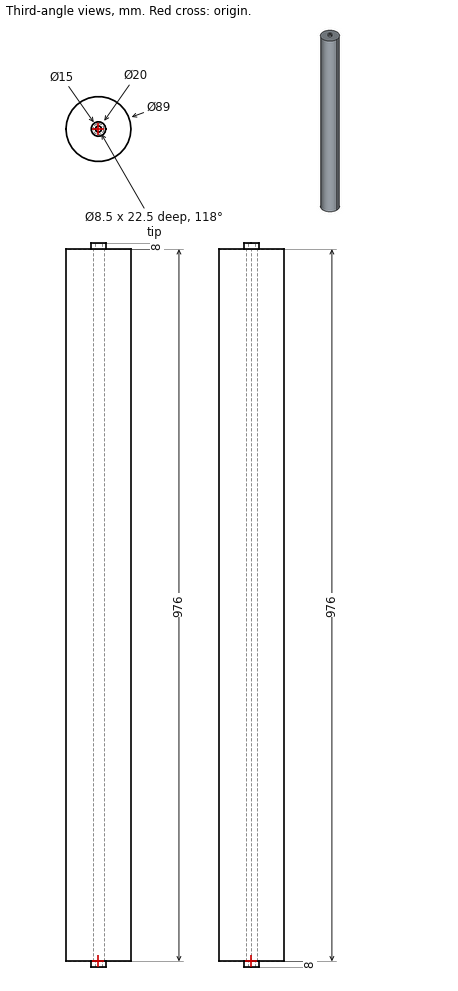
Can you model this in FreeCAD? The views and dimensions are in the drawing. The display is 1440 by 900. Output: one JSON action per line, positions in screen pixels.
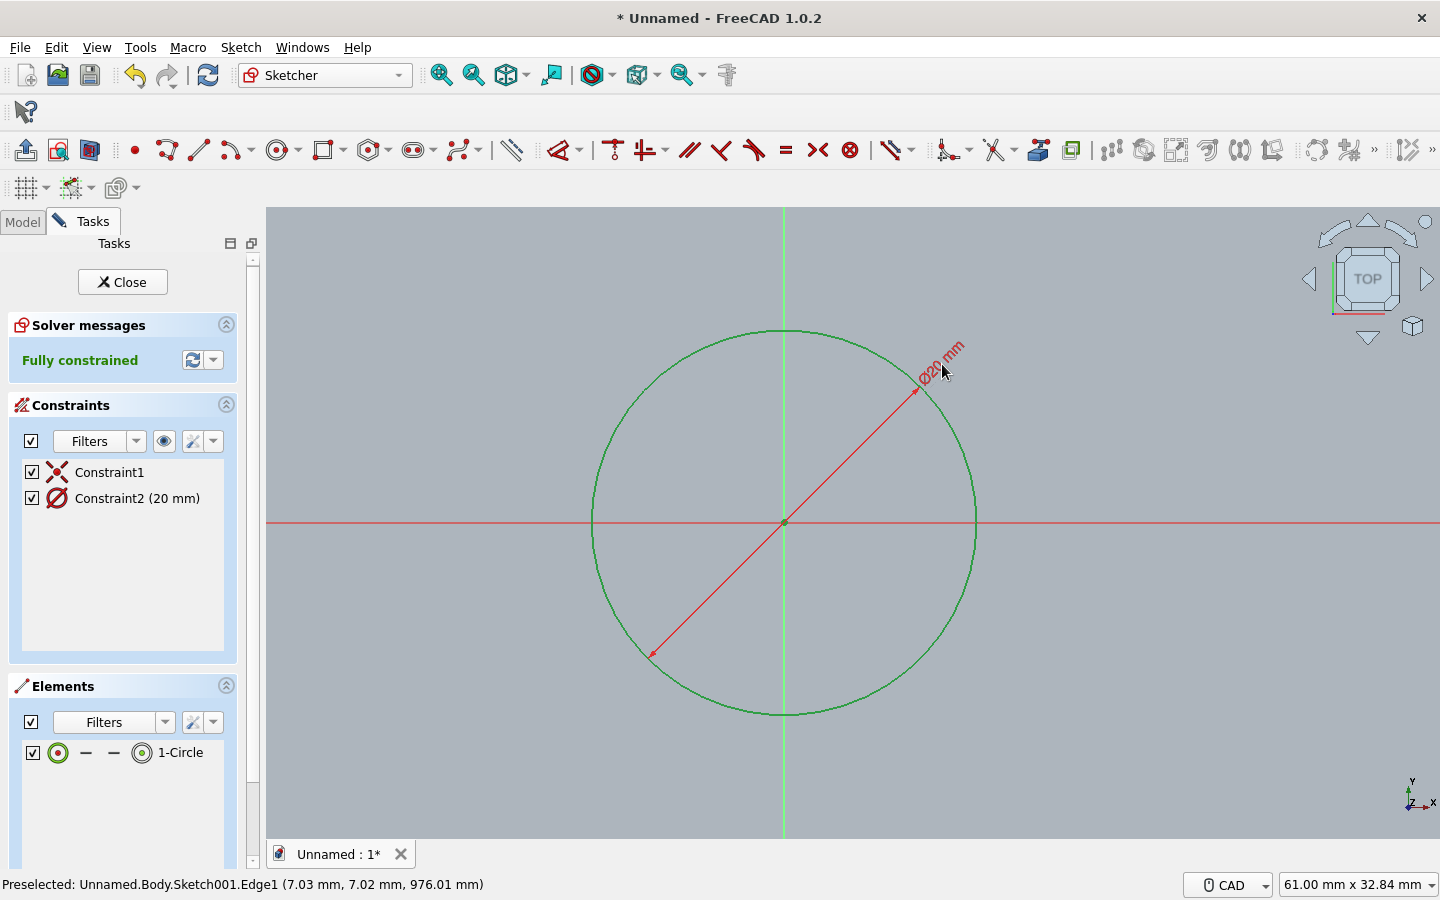
{"action": "left_click", "coordinate": [123, 282]}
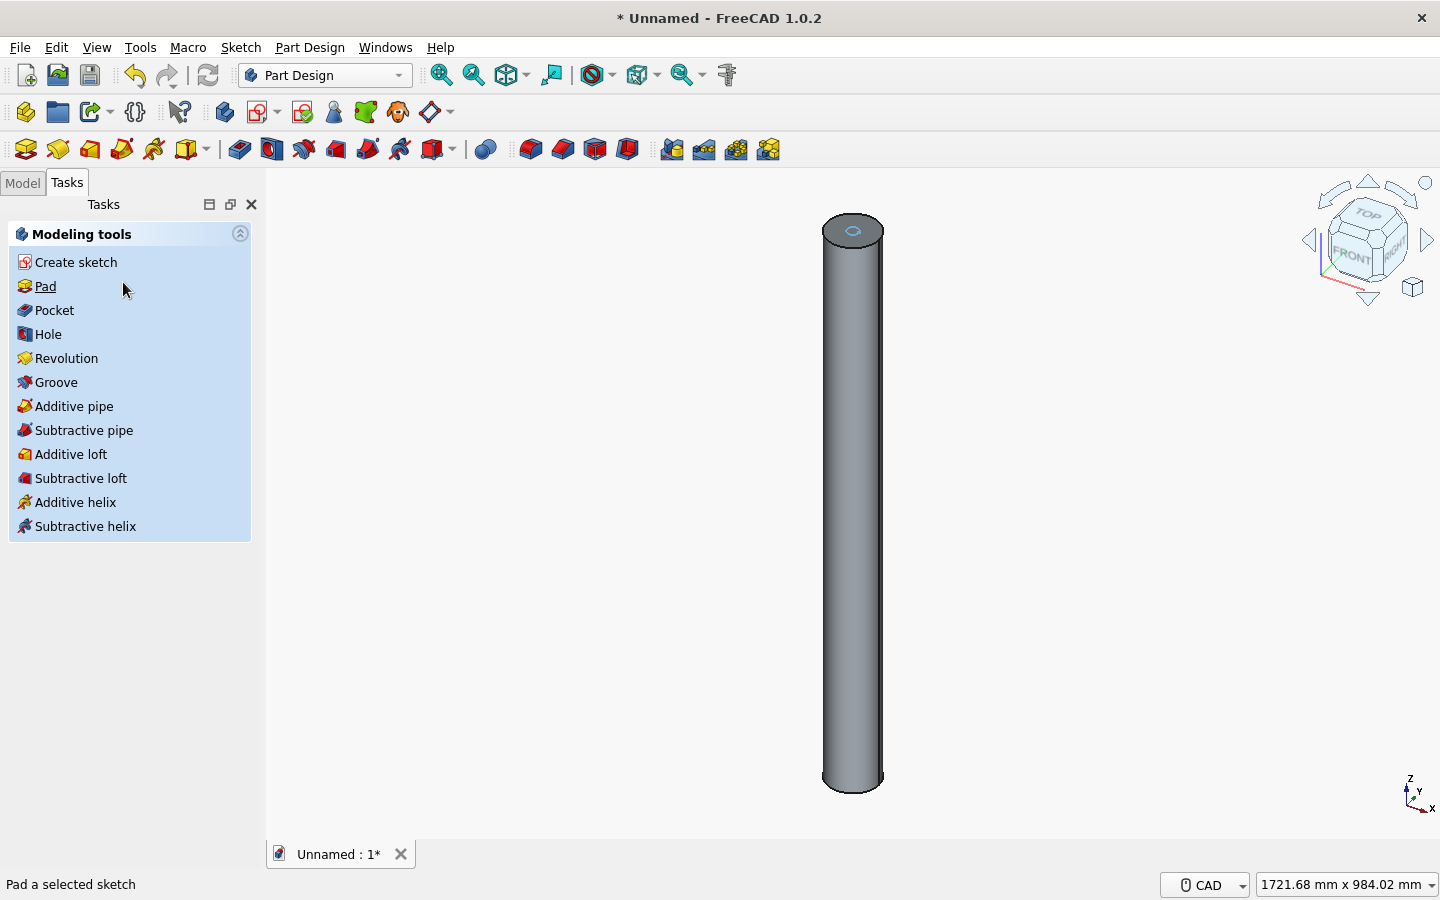
{"action": "left_click", "coordinate": [26, 150]}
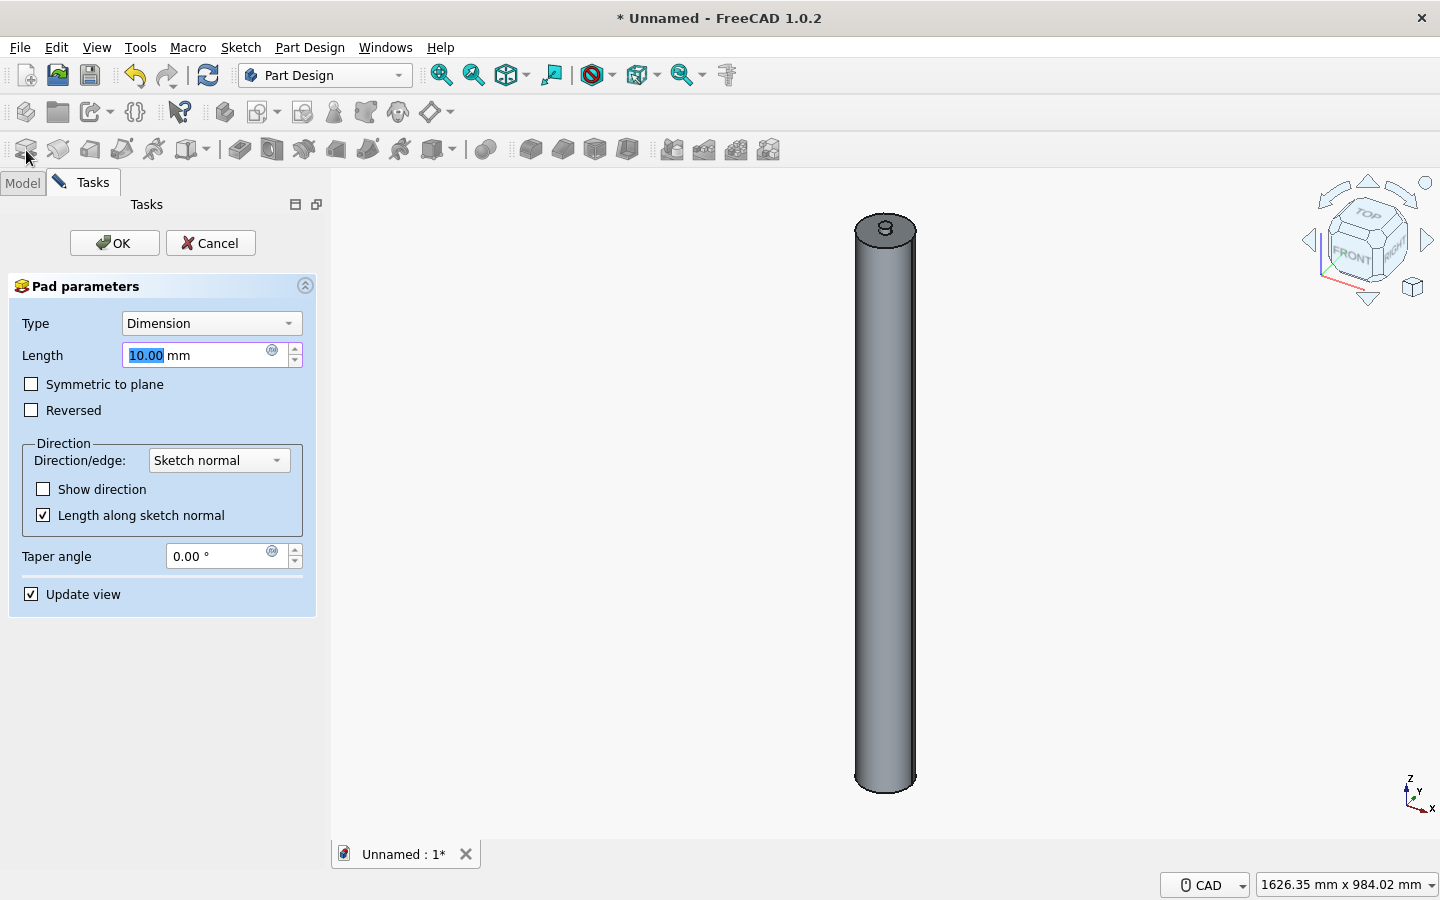
{"action": "type", "text": "8"}
{"action": "key", "text": "Tab"}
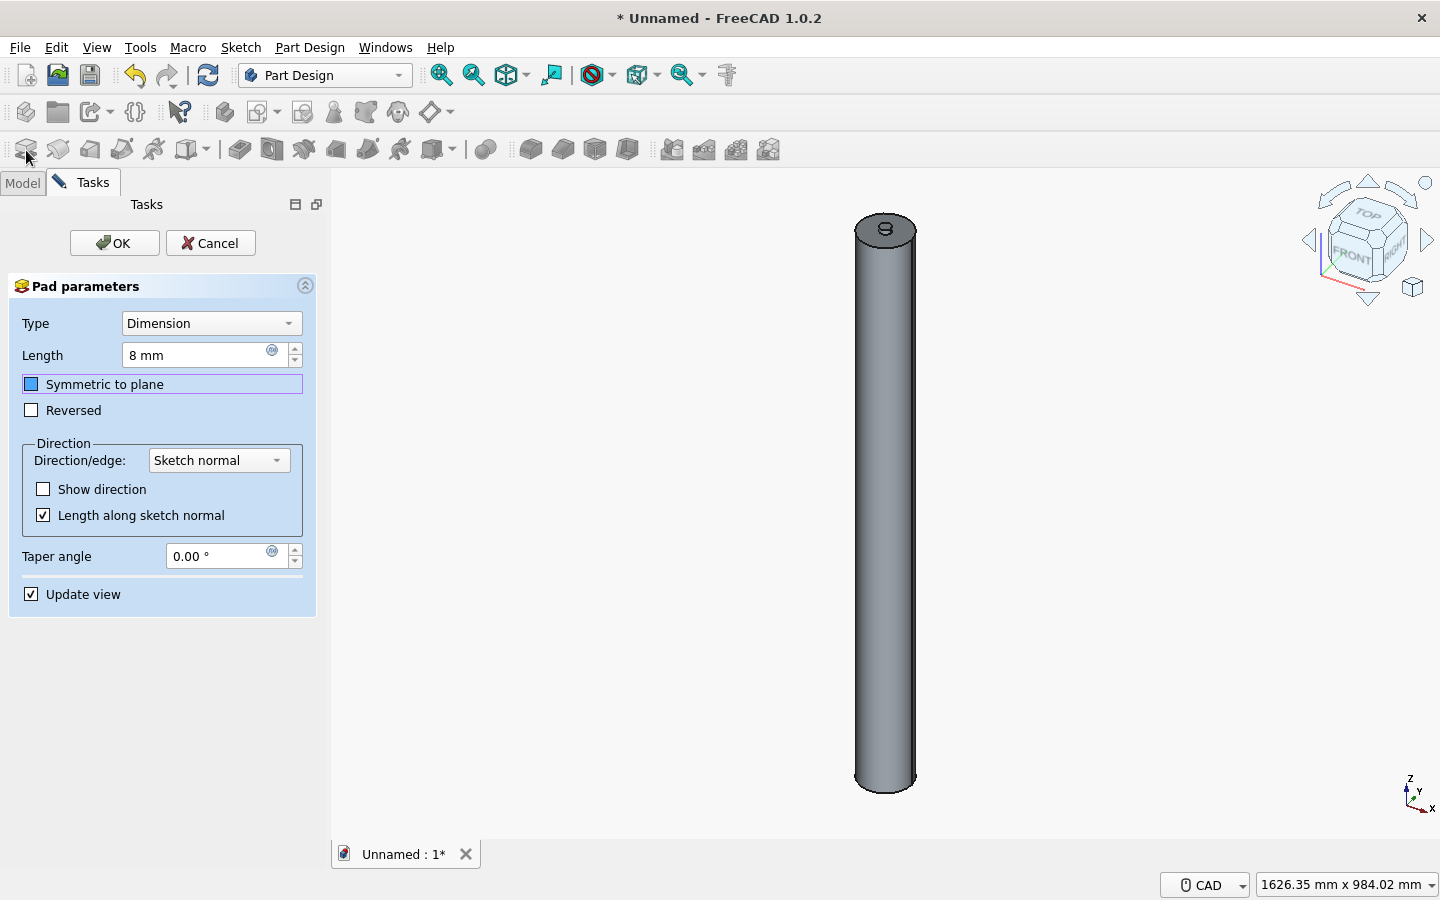
{"action": "left_click", "coordinate": [115, 243]}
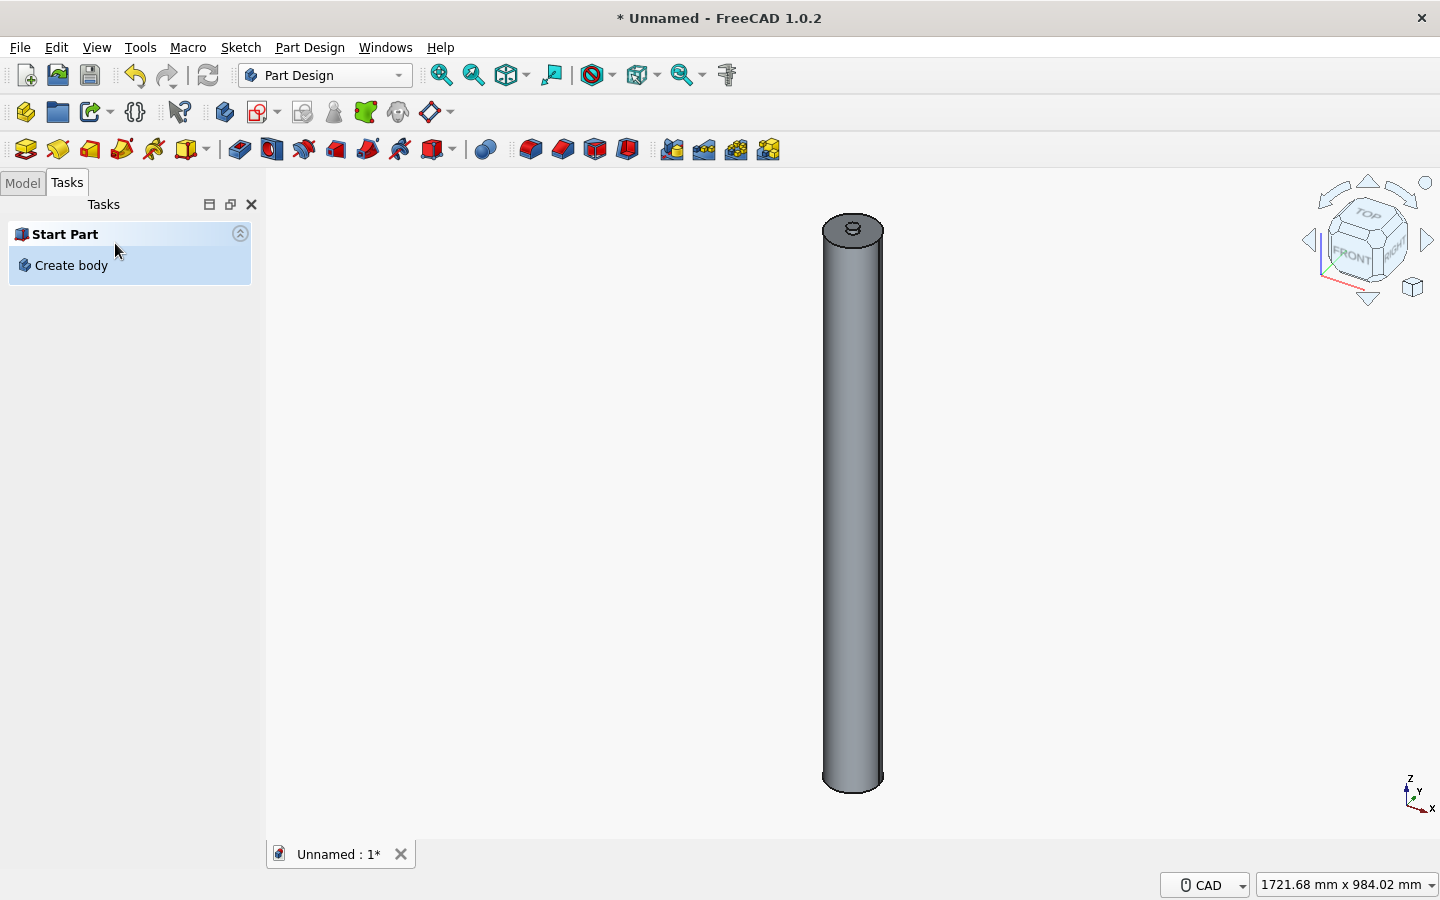
{"action": "left_click", "coordinate": [23, 182]}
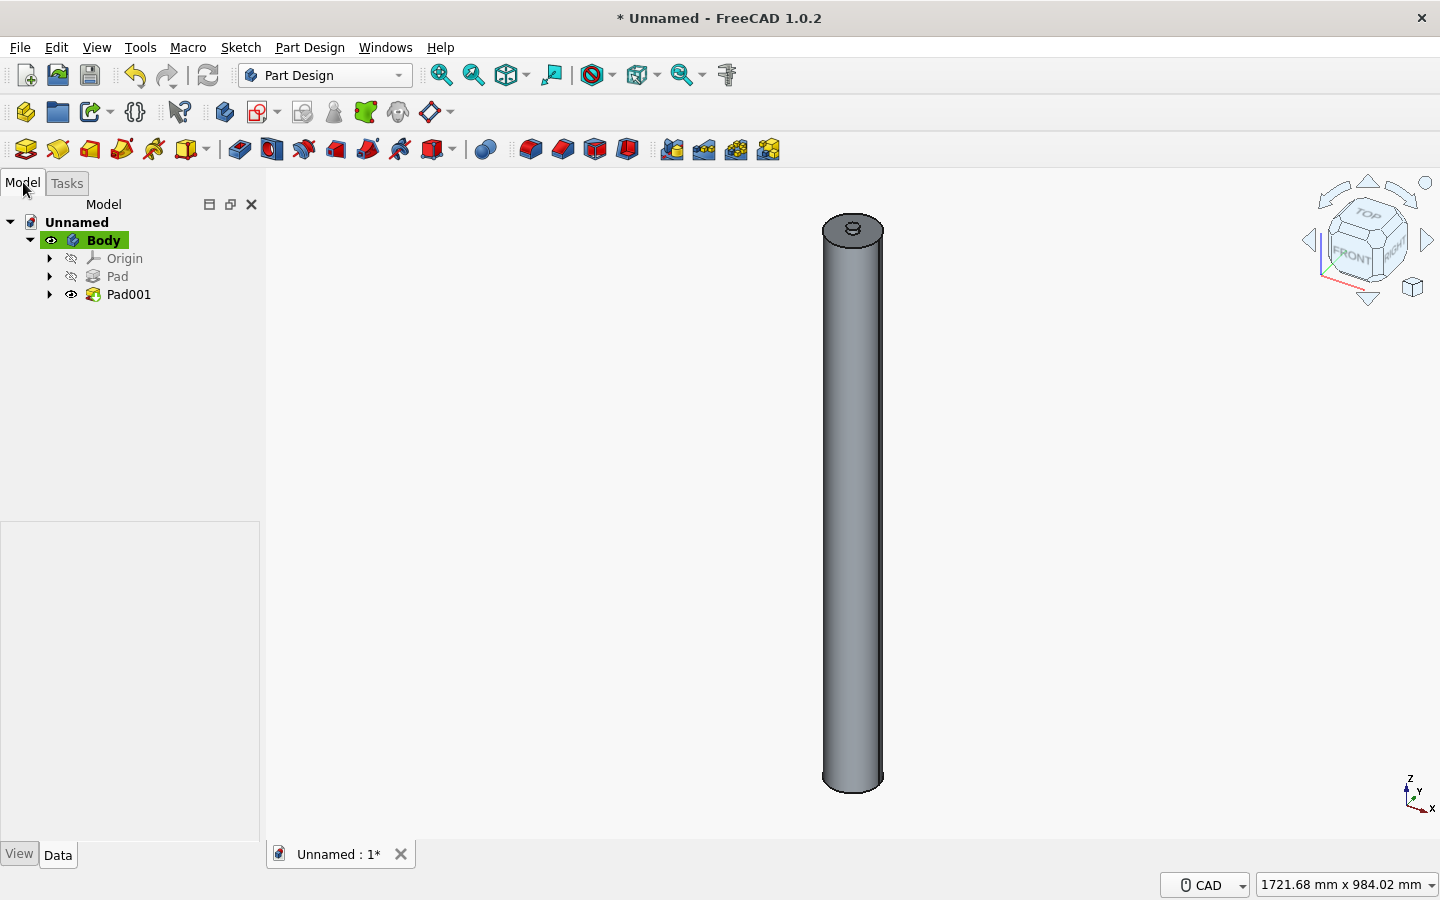
{"action": "left_click", "coordinate": [50, 258]}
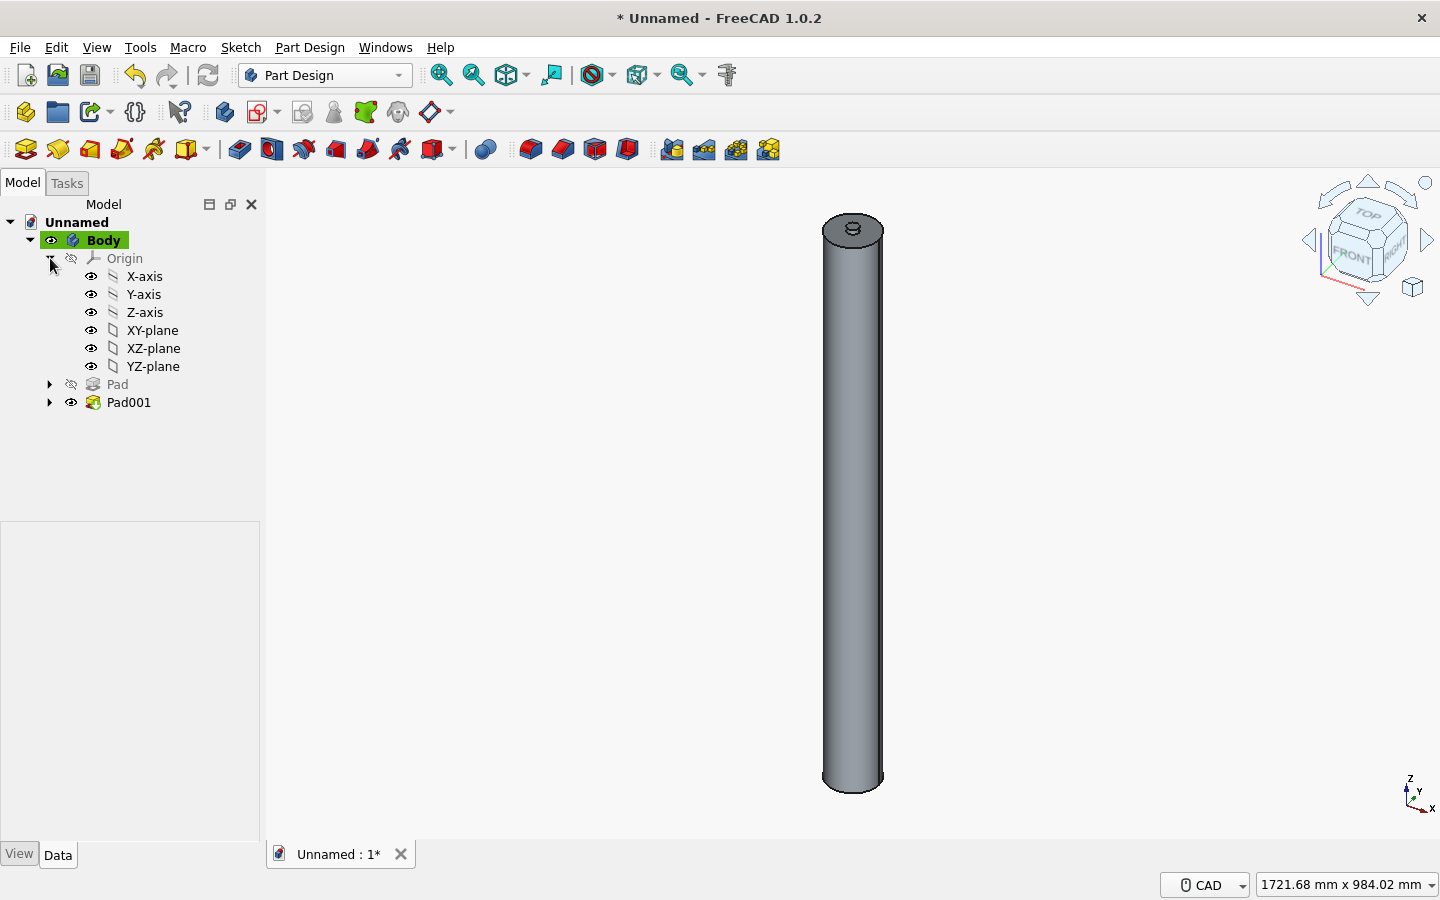
{"action": "left_click", "coordinate": [136, 330]}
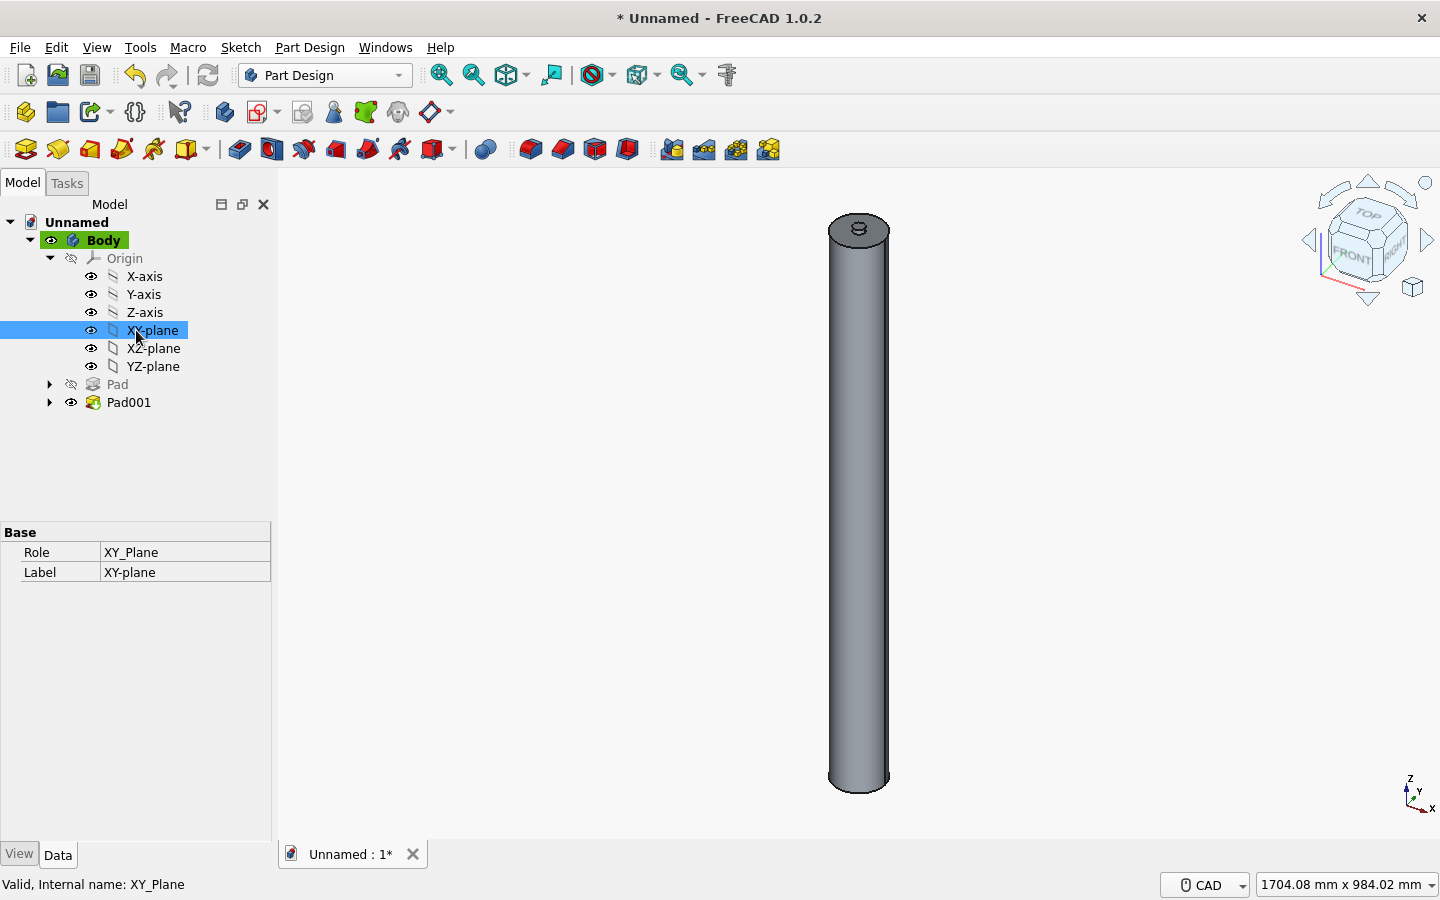
{"action": "left_click", "coordinate": [430, 112]}